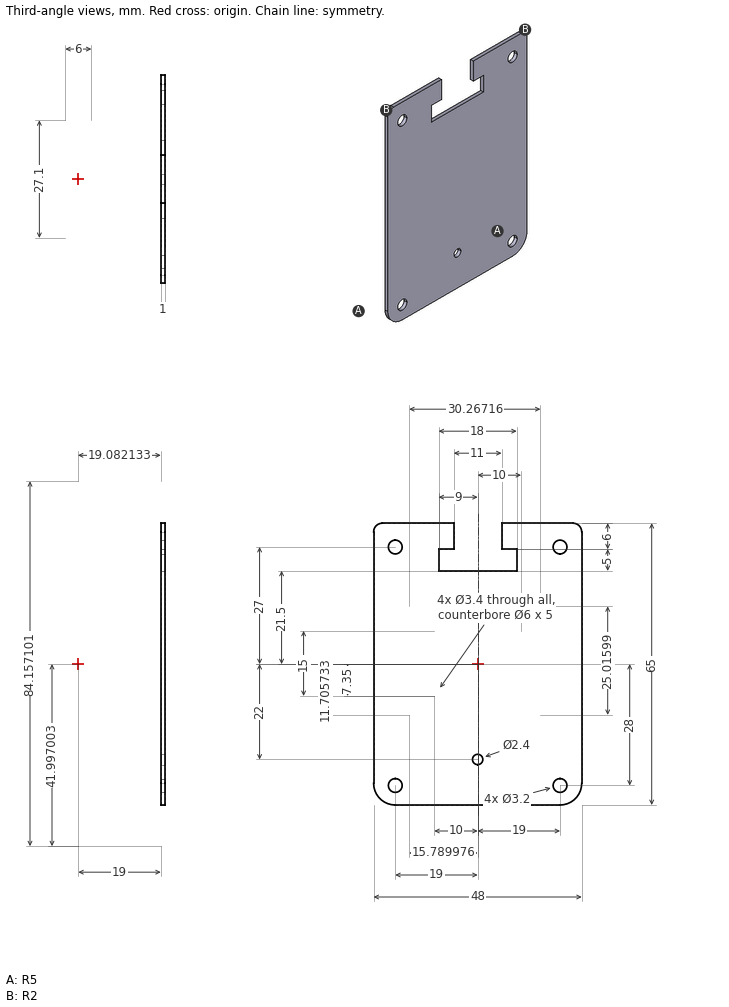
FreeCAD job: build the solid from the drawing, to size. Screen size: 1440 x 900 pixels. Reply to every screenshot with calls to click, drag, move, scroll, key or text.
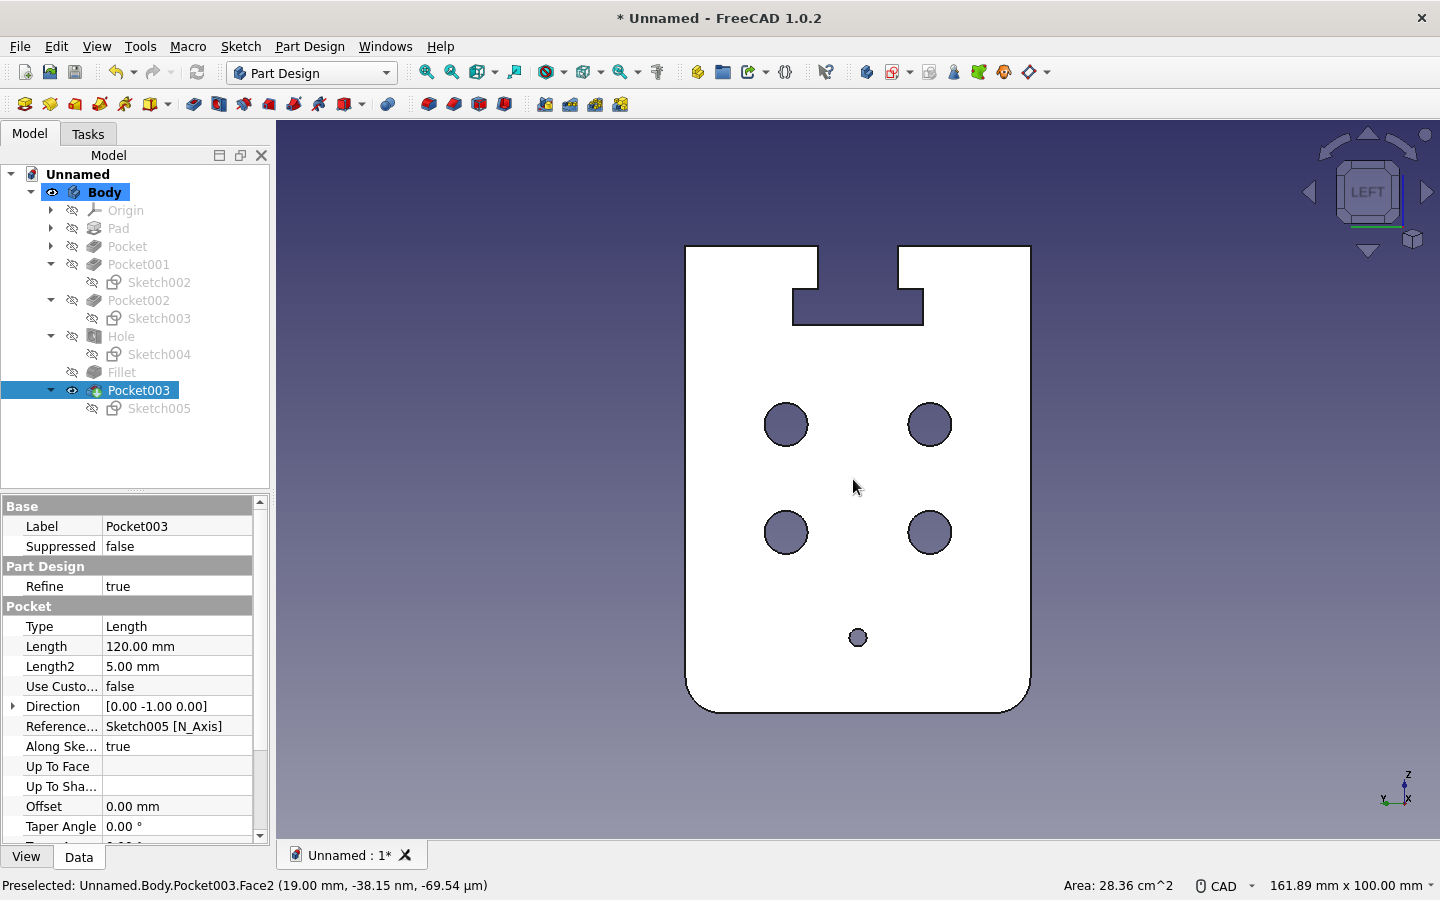
click(892, 72)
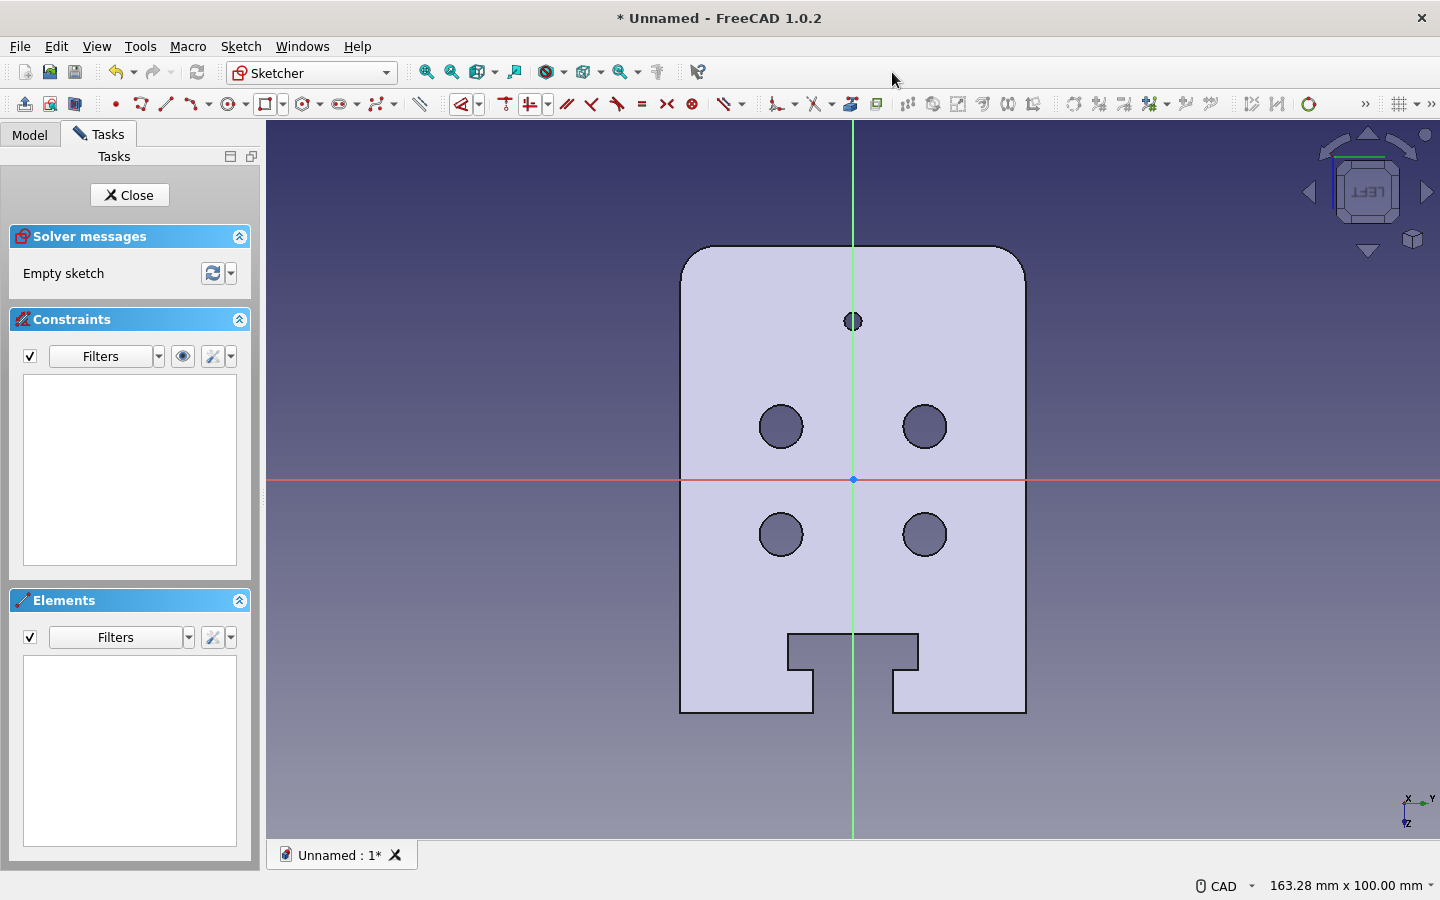
scroll(885, 489, up, 5)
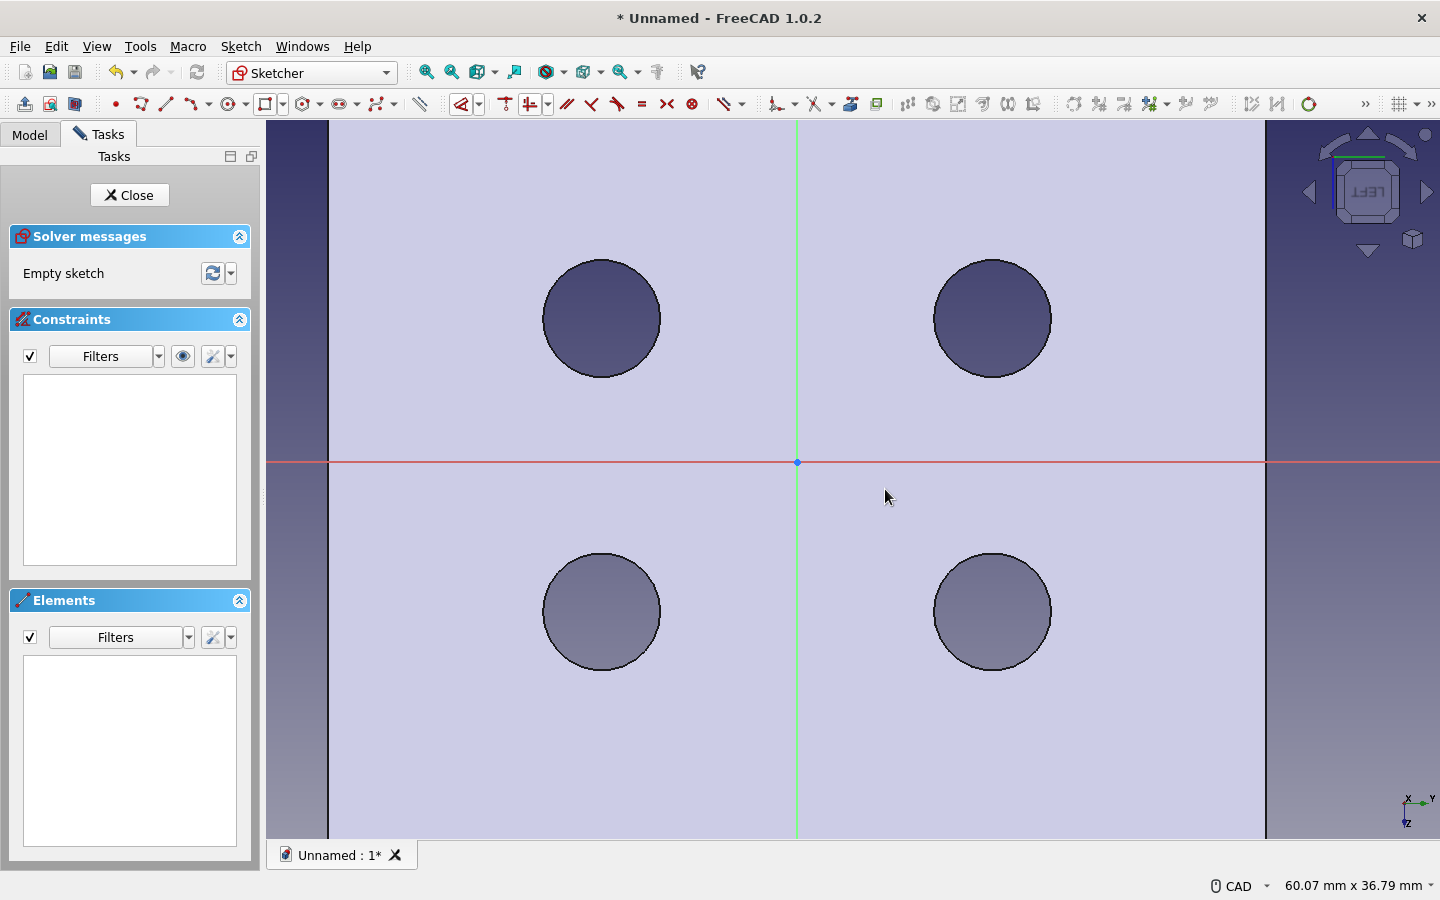
key(g)
key(r)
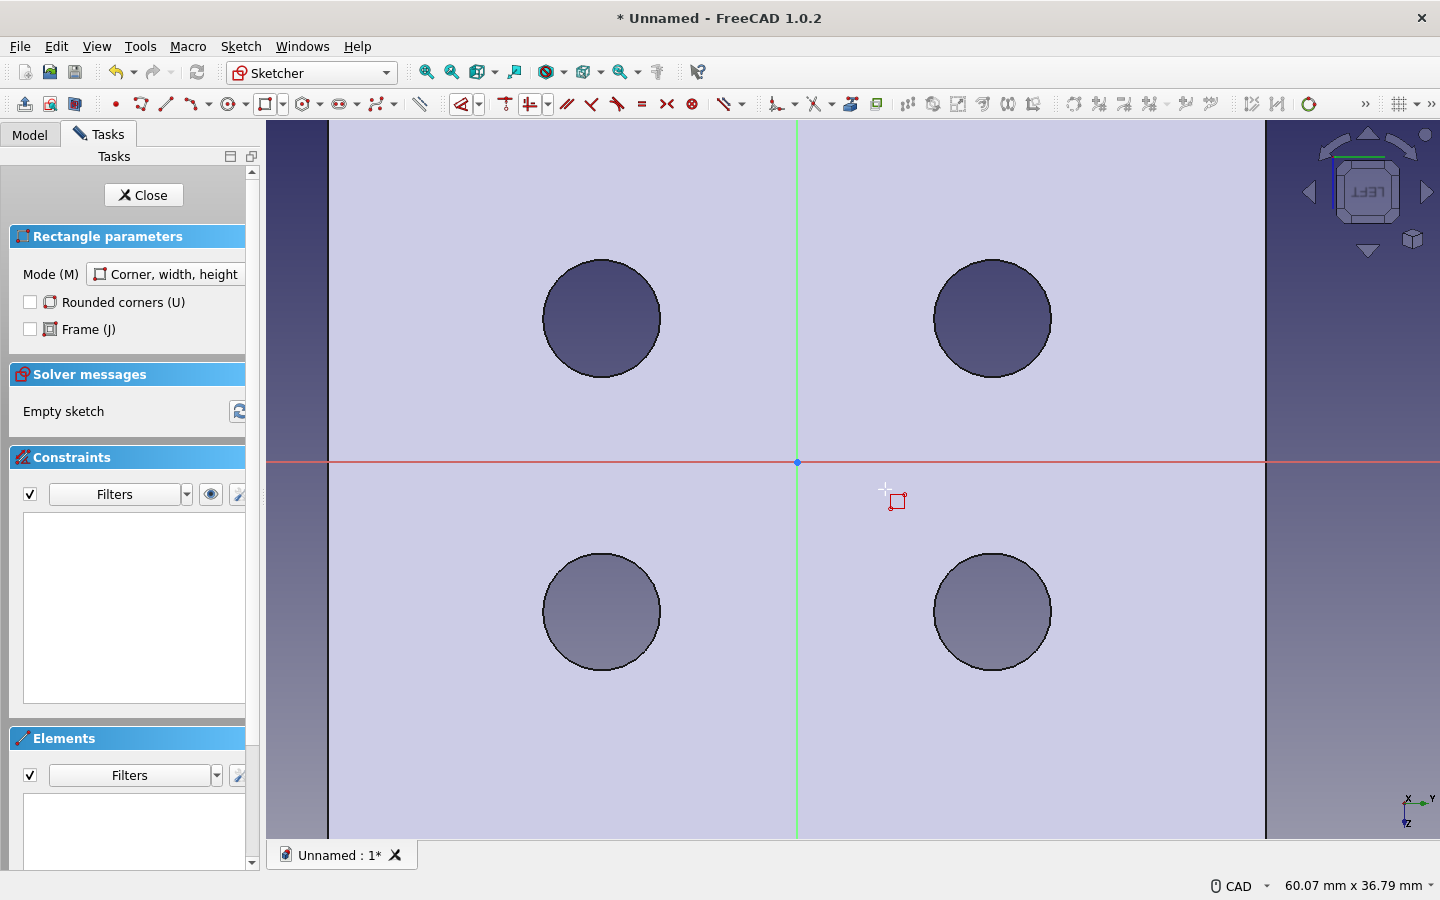
click(489, 234)
move(1080, 722)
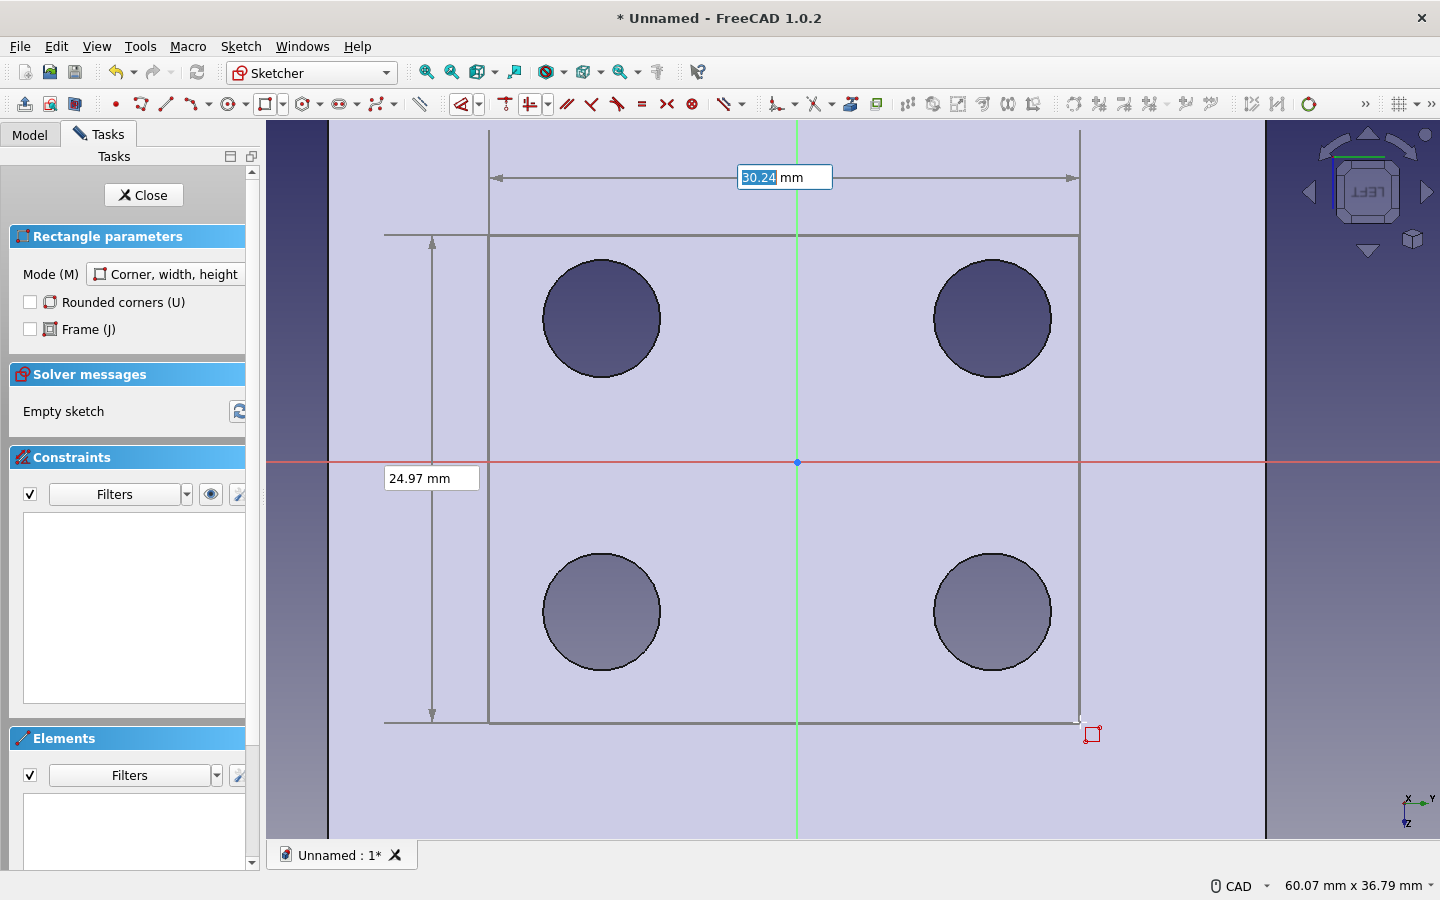
text(30.26716)
key(Tab)
text(25.01599)
key(Return)
key(Escape)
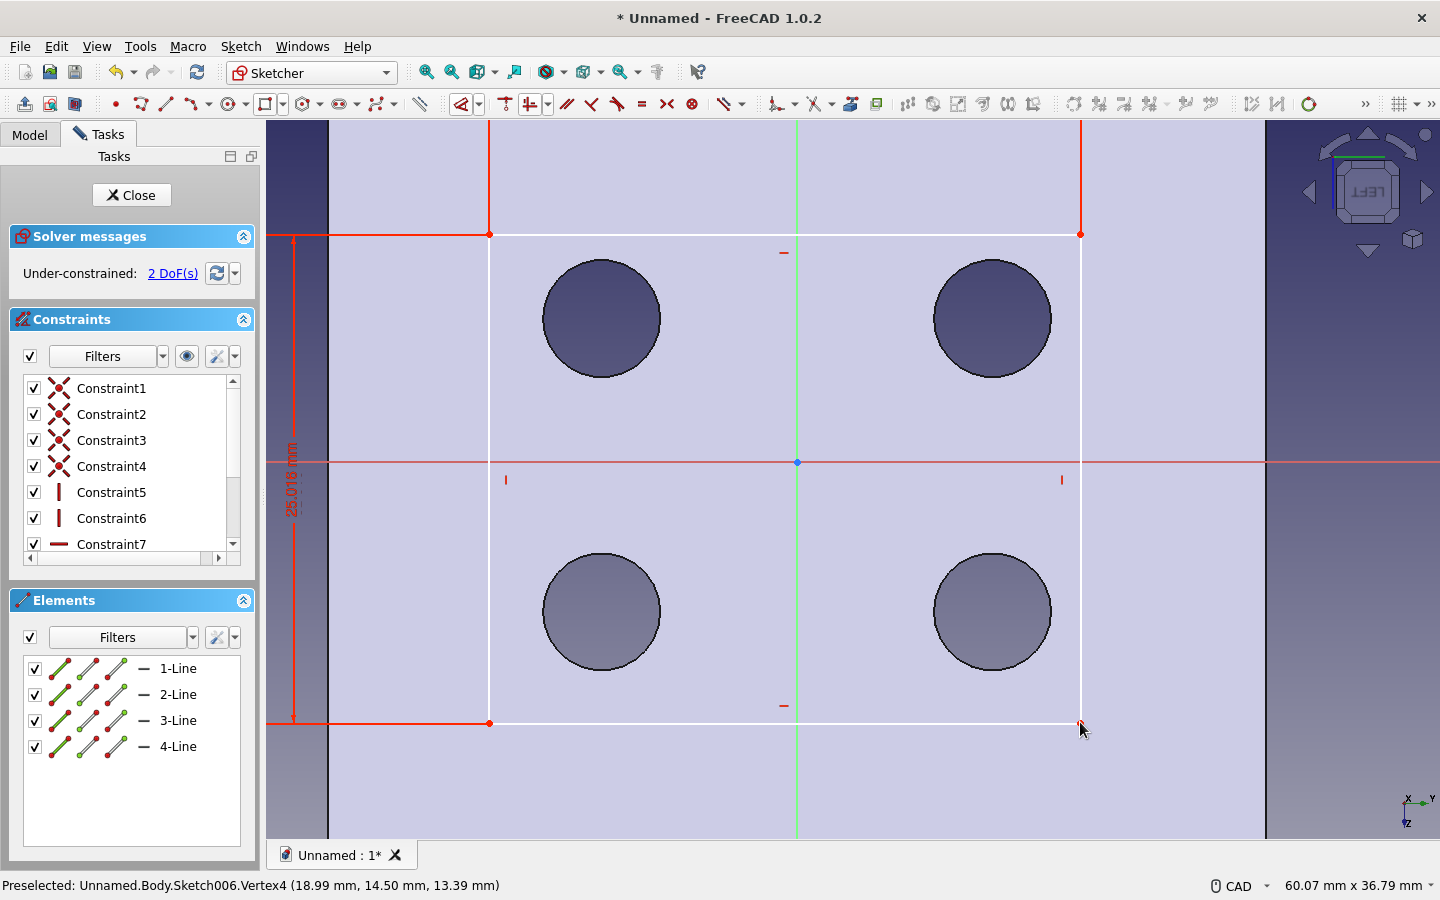
click(489, 235)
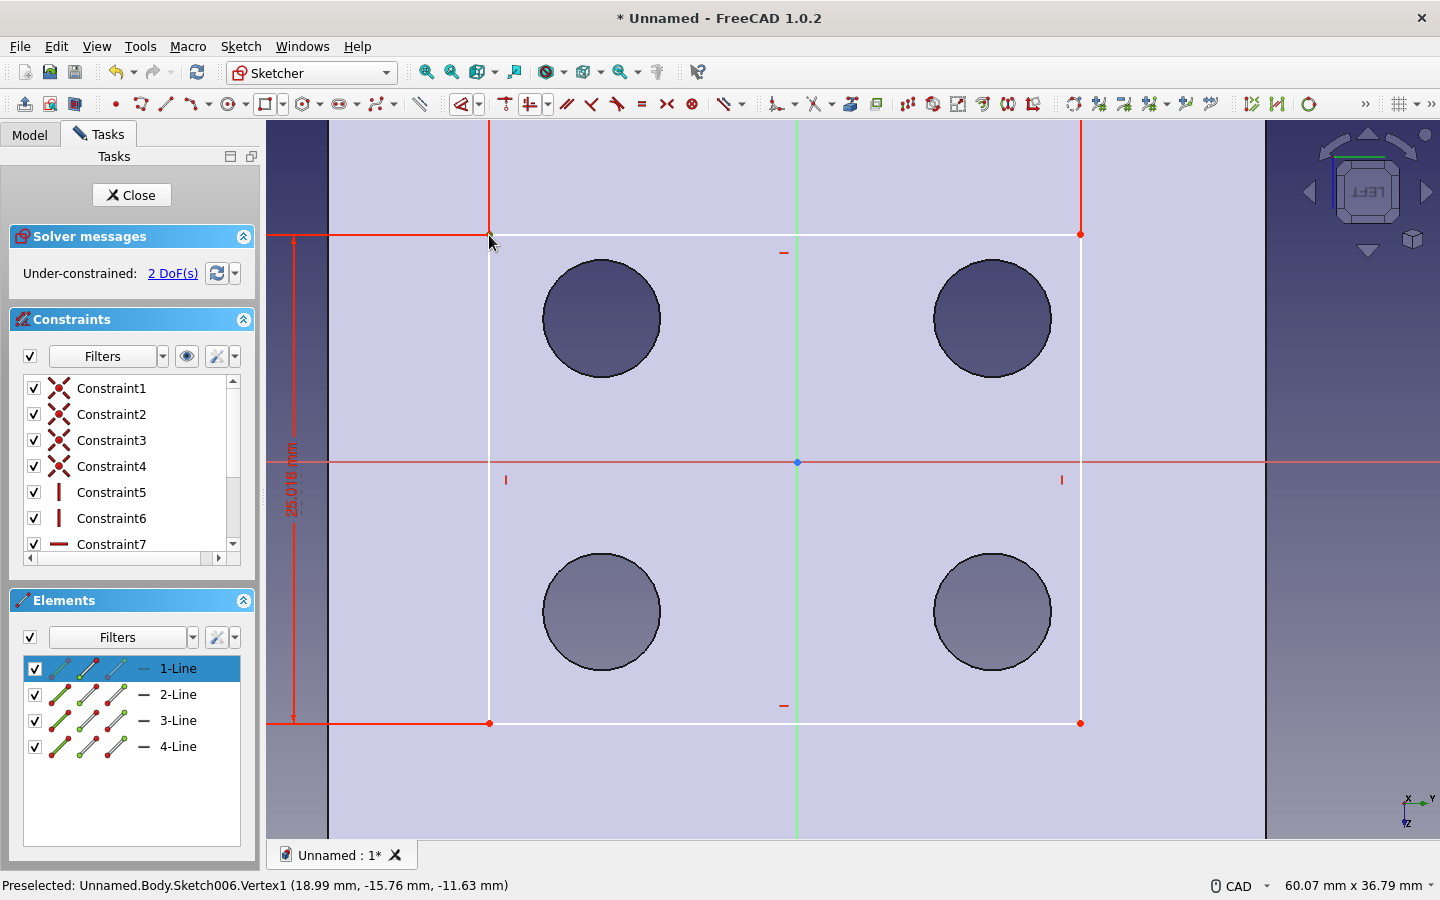
key(l)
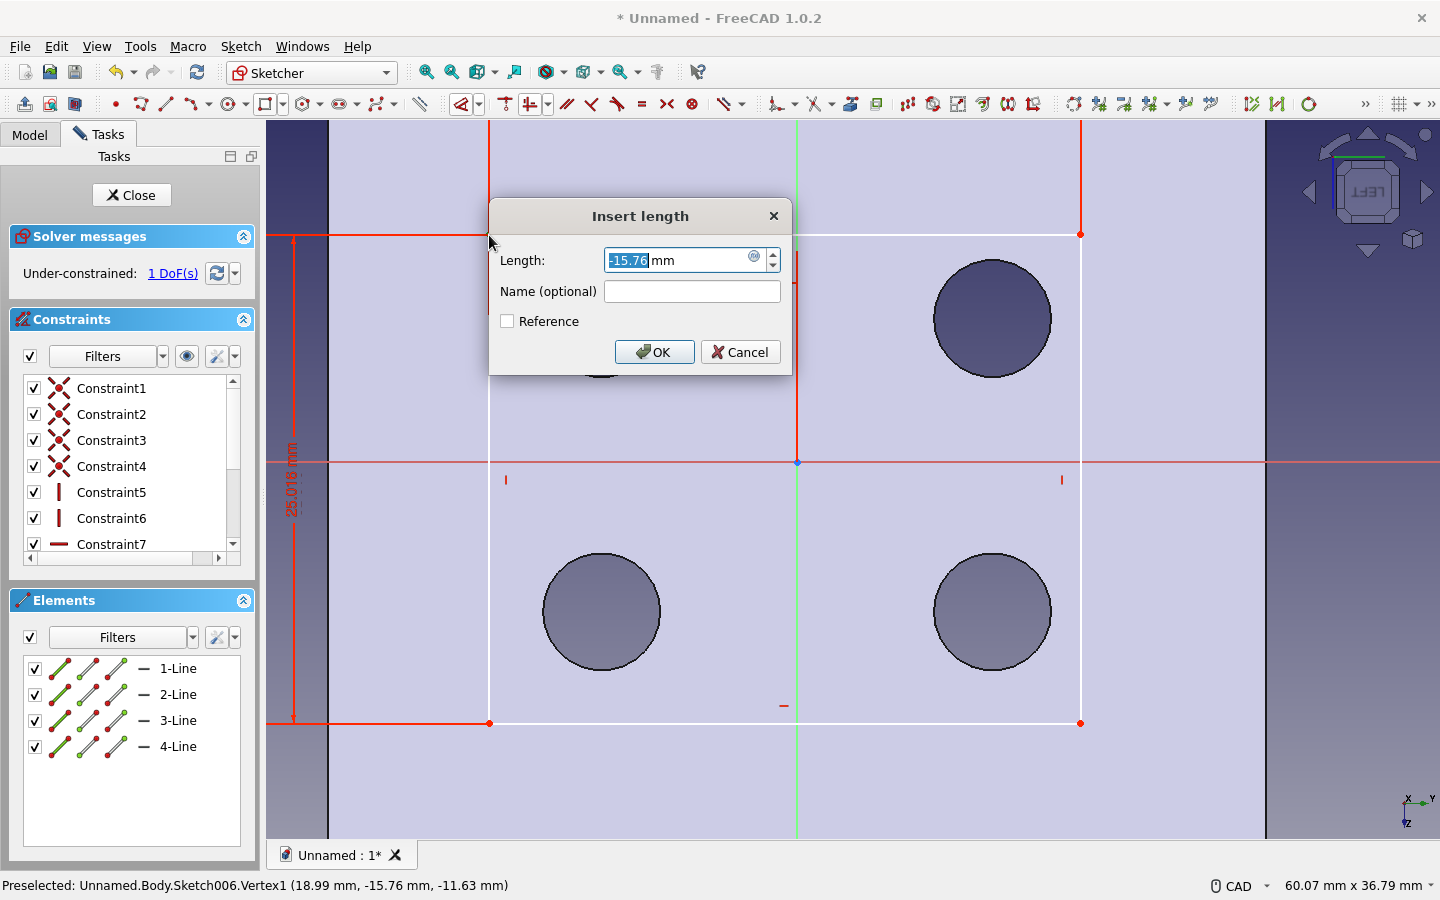
text(-15.789976)
key(Return)